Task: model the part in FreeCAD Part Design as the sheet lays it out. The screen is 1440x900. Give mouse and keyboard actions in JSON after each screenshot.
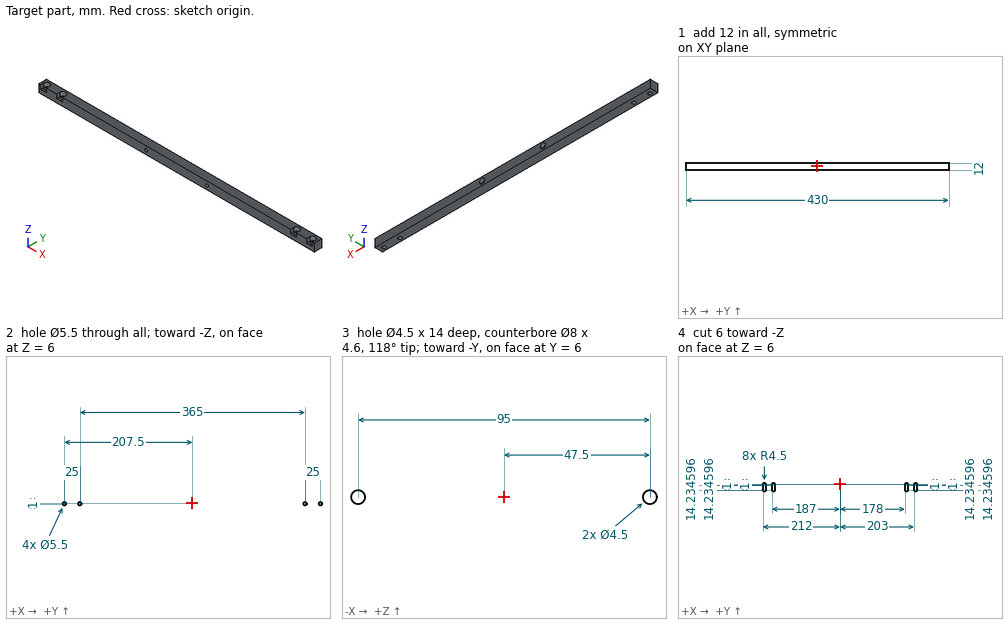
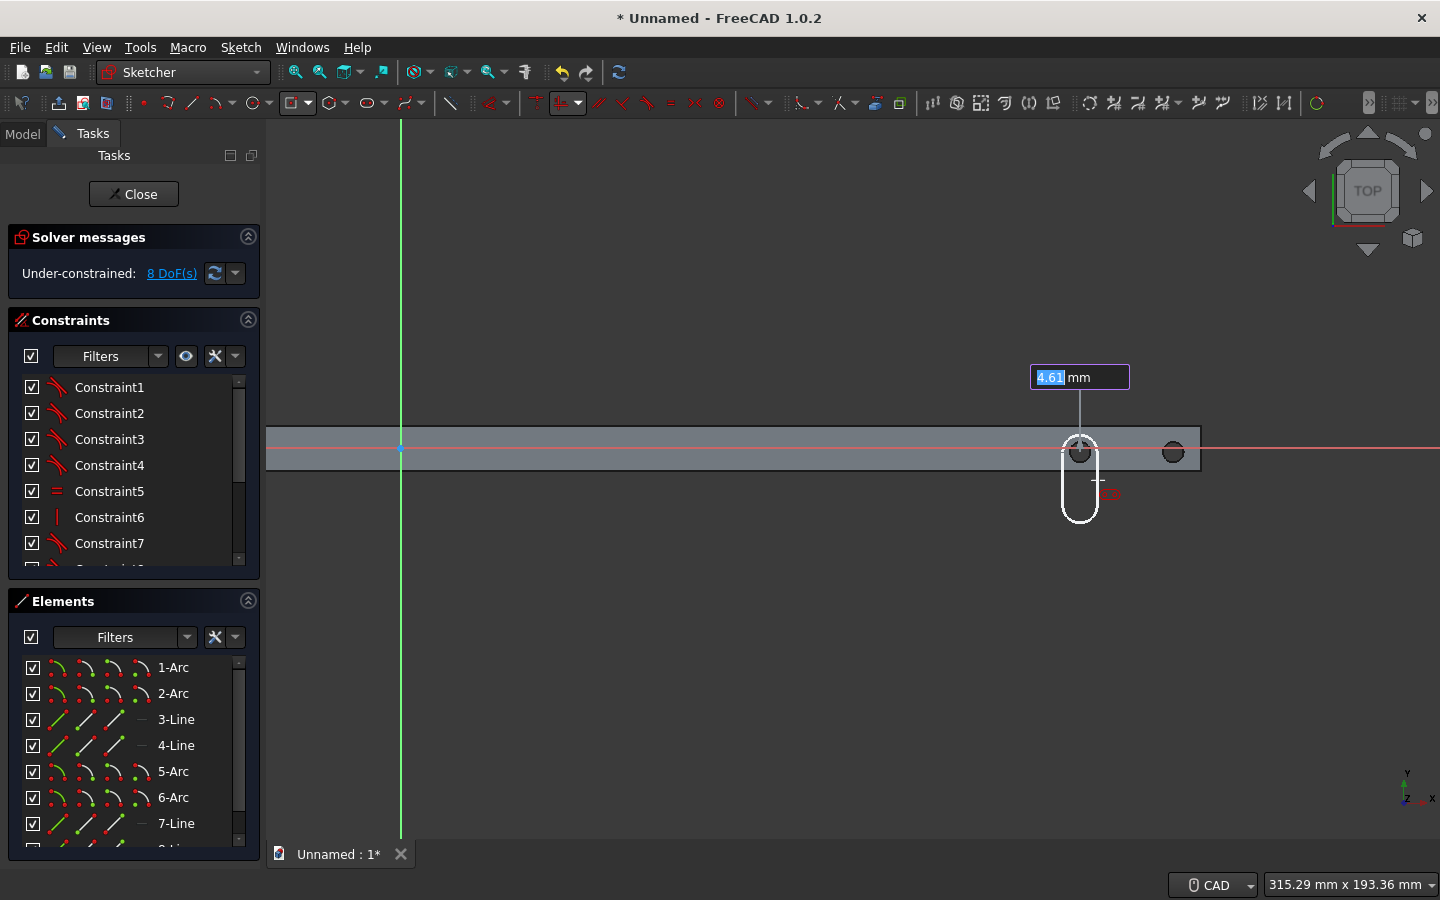
{"action": "left_click", "coordinate": [1097, 479]}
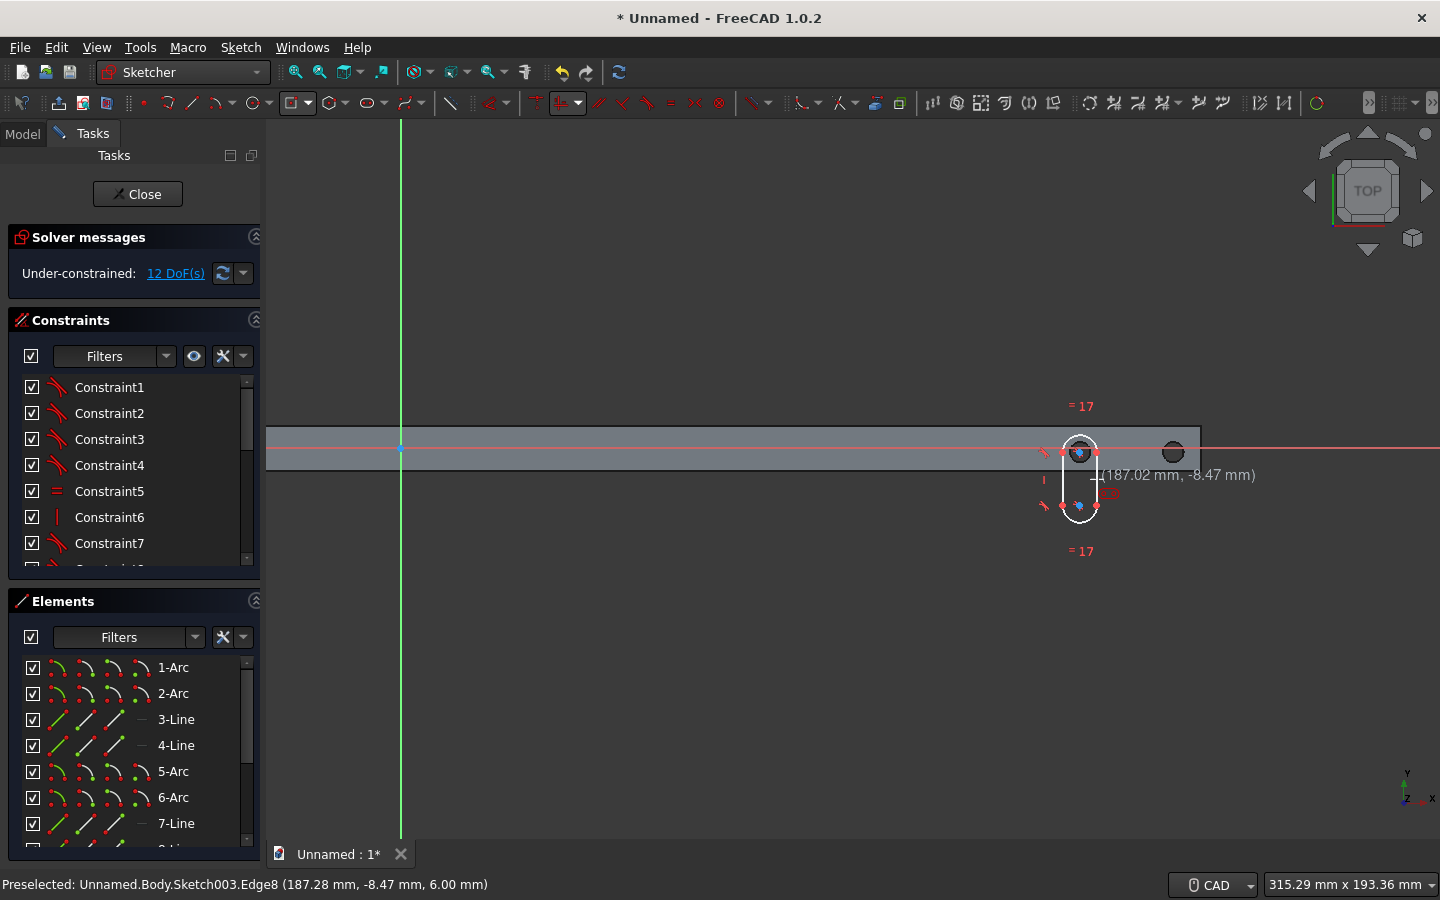
{"action": "scroll", "coordinate": [1173, 505], "scroll_direction": "up", "scroll_amount": 2}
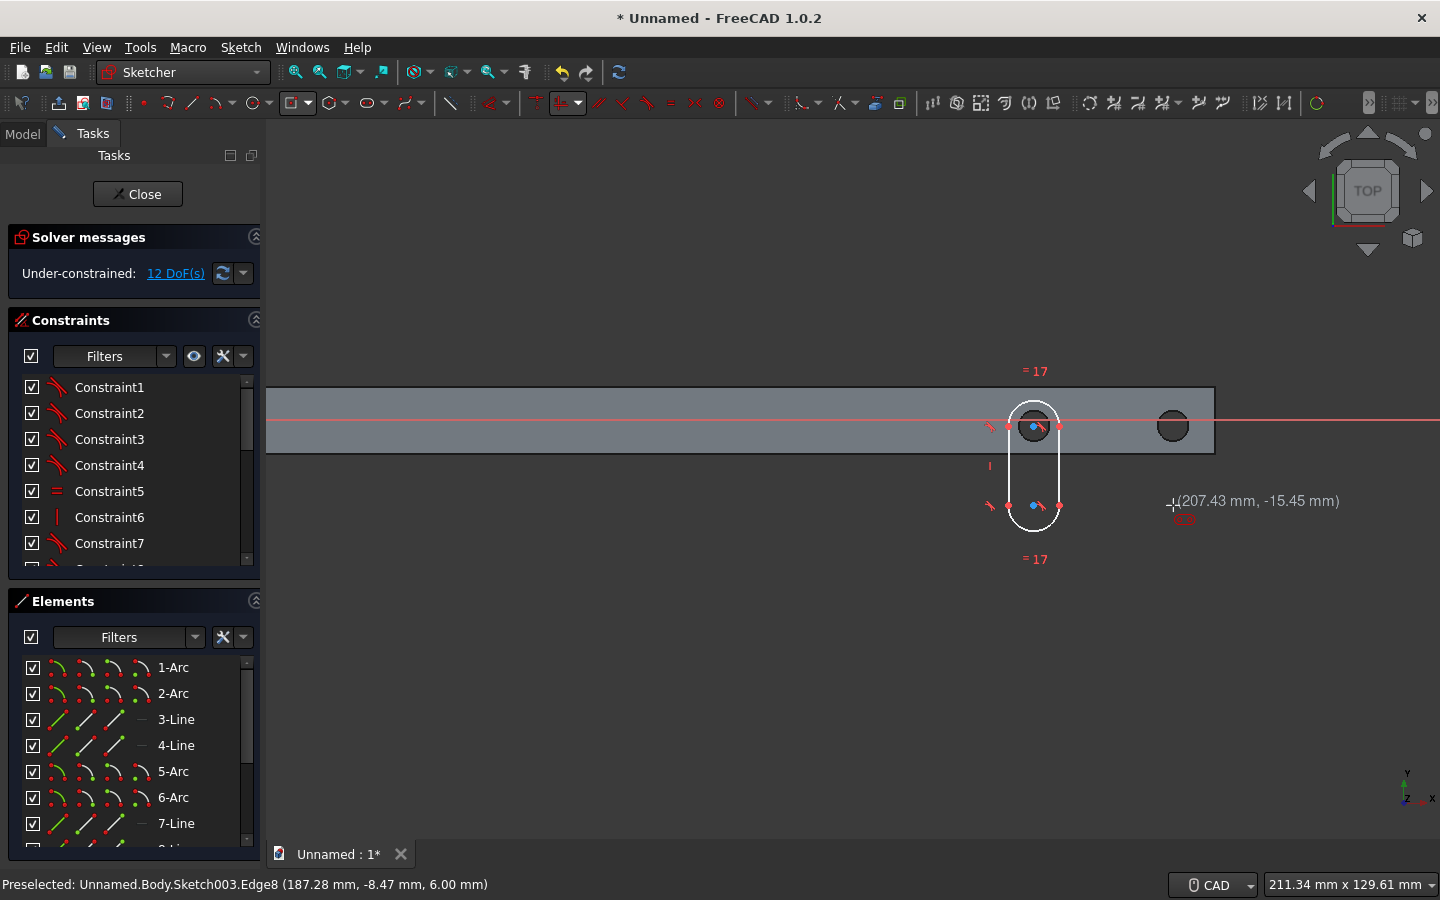
{"action": "left_click", "coordinate": [1173, 505]}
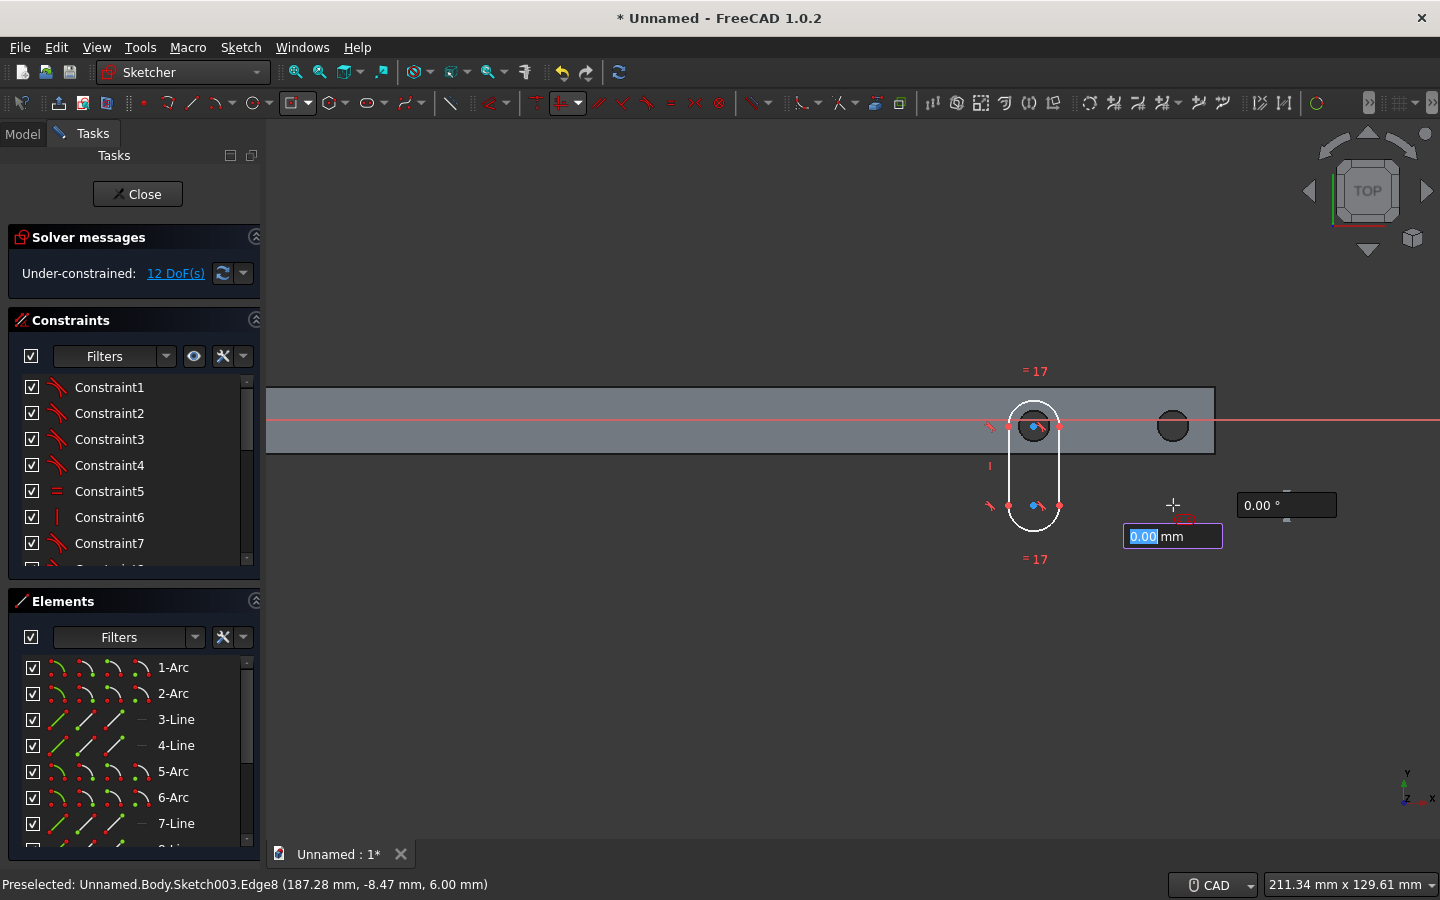
{"action": "scroll", "coordinate": [1173, 426], "scroll_direction": "up", "scroll_amount": 6}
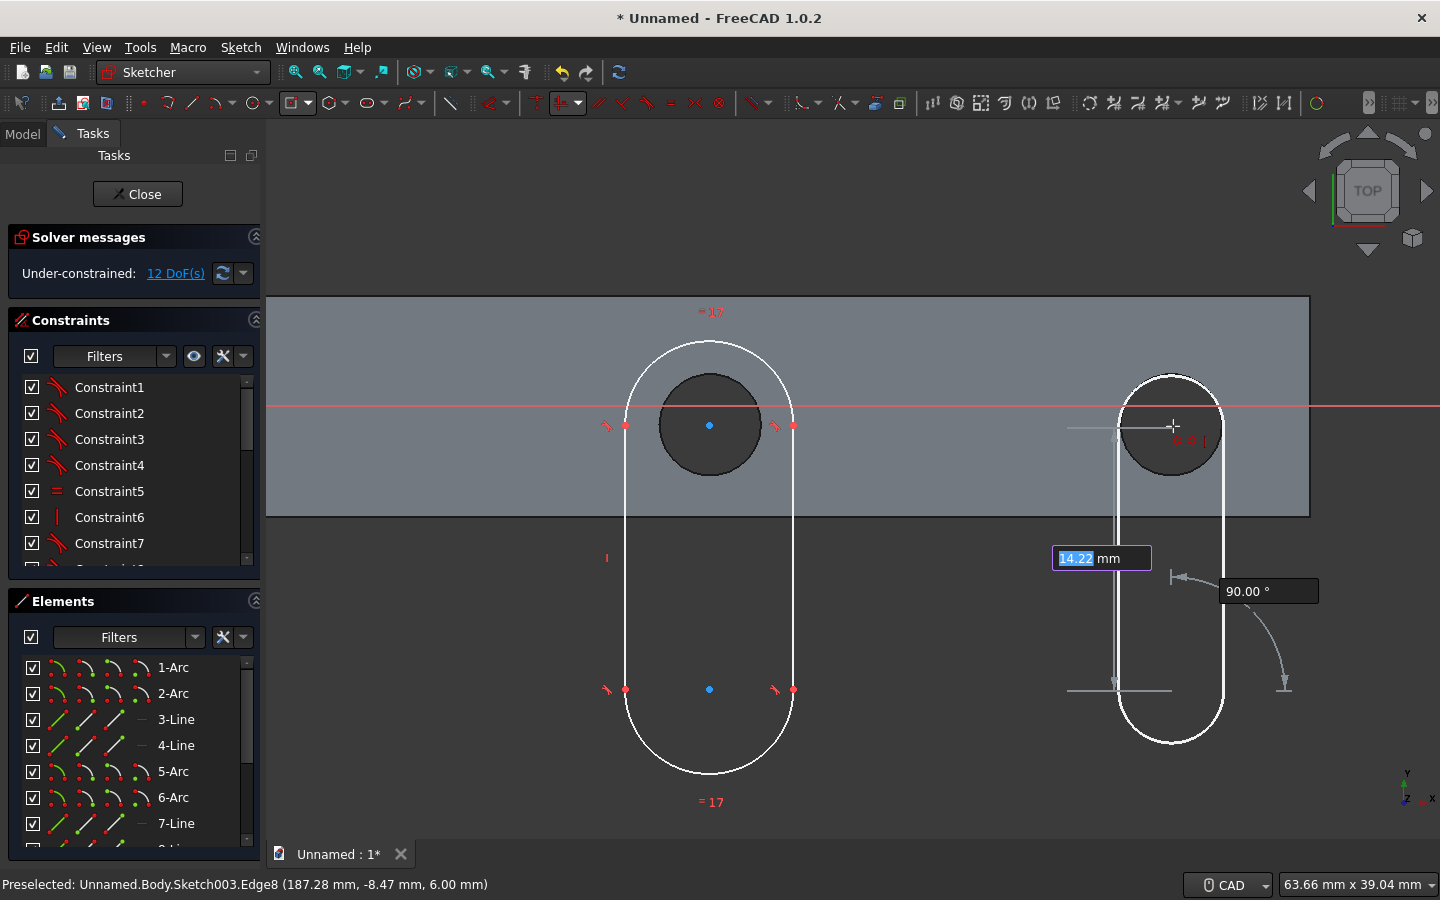
{"action": "left_click", "coordinate": [1171, 425]}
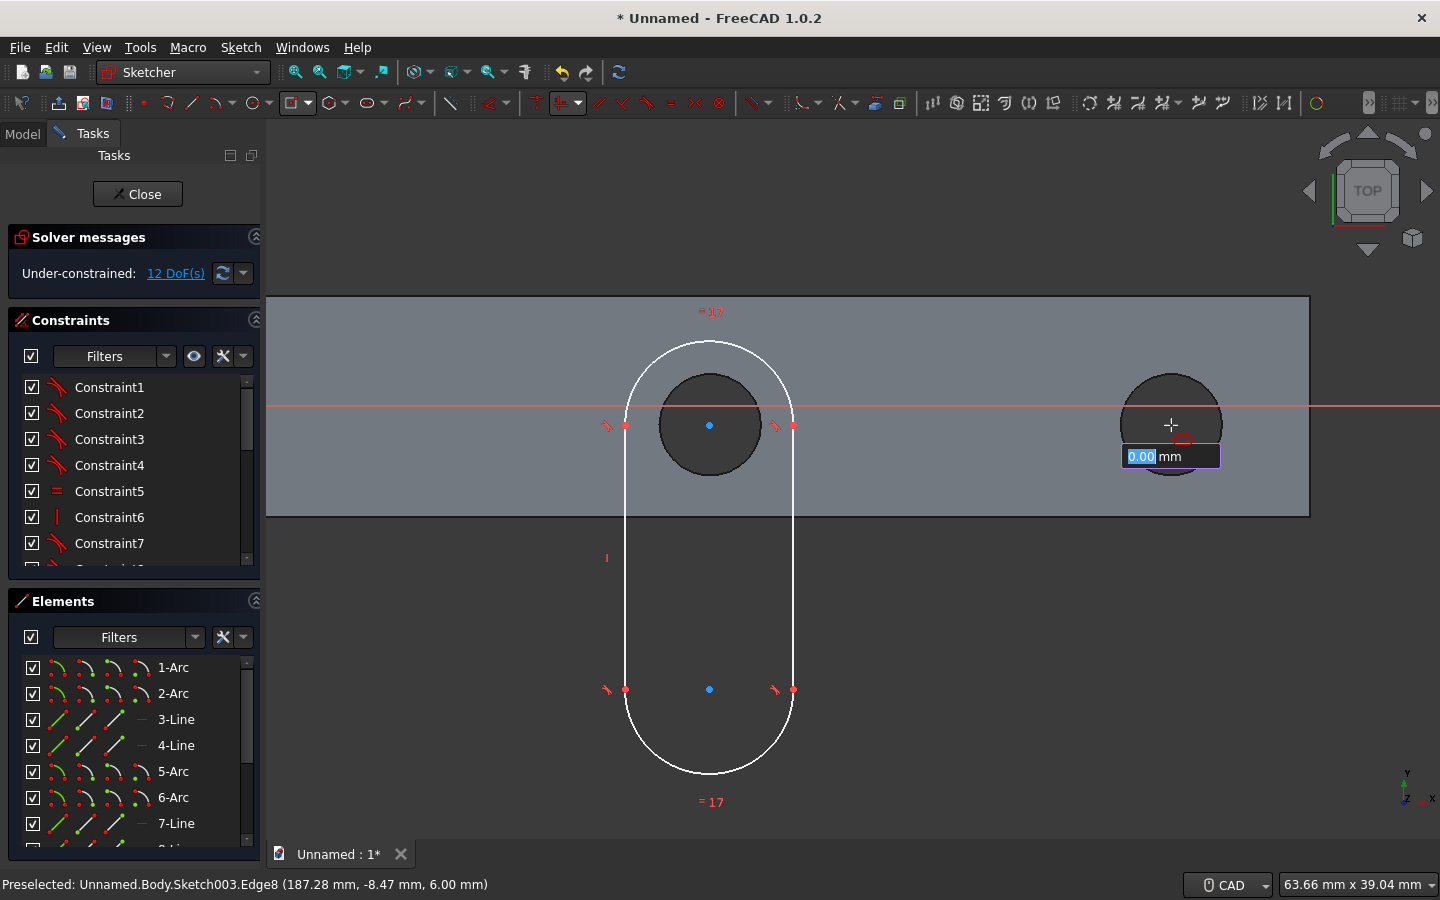
{"action": "scroll", "coordinate": [1128, 471], "scroll_direction": "down", "scroll_amount": 12}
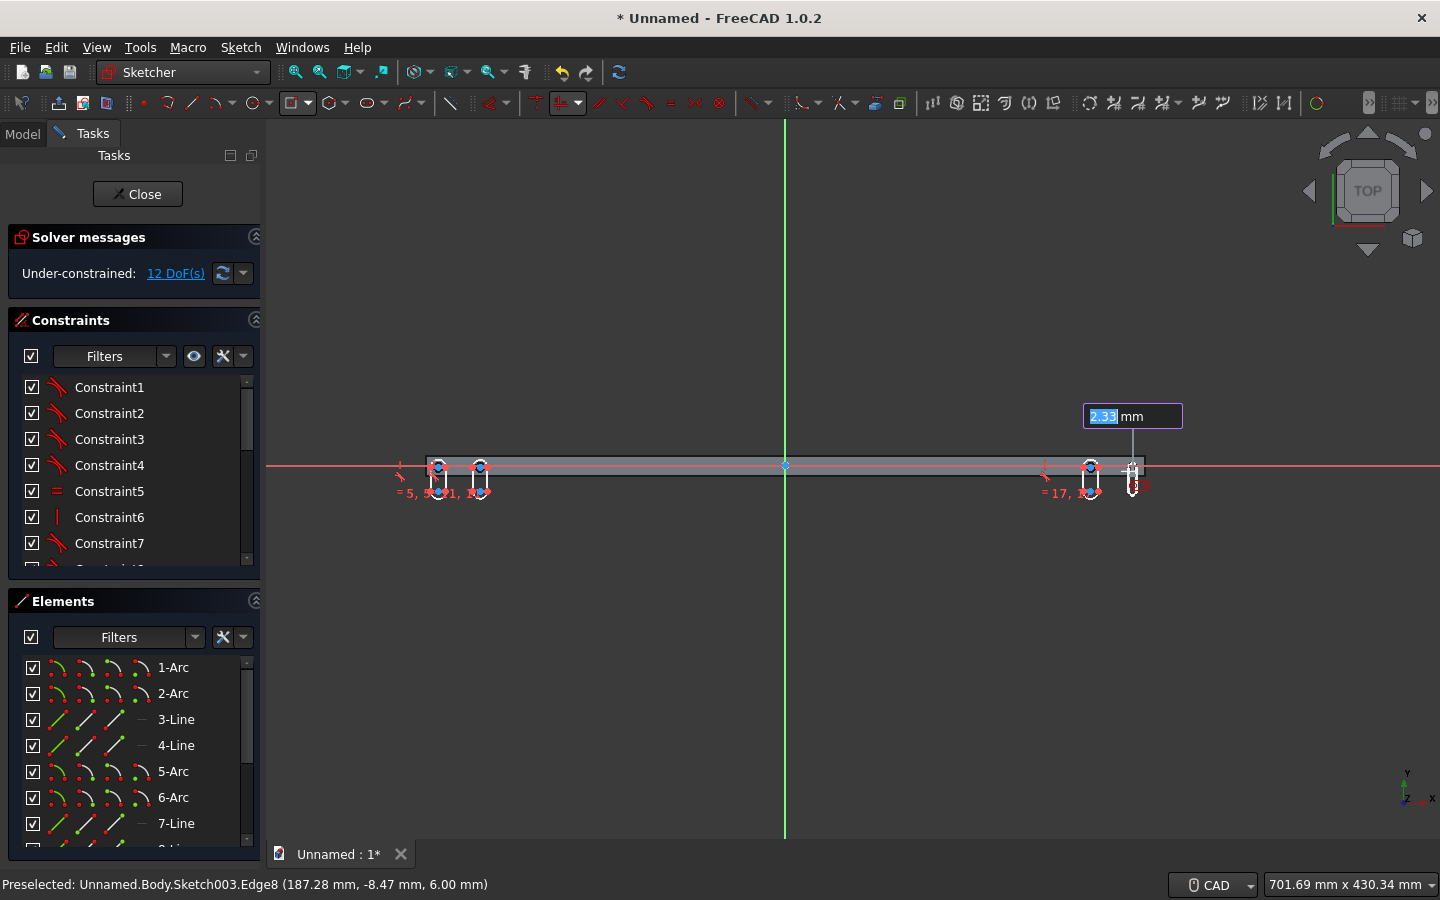
{"action": "scroll", "coordinate": [1140, 479], "scroll_direction": "up", "scroll_amount": 4}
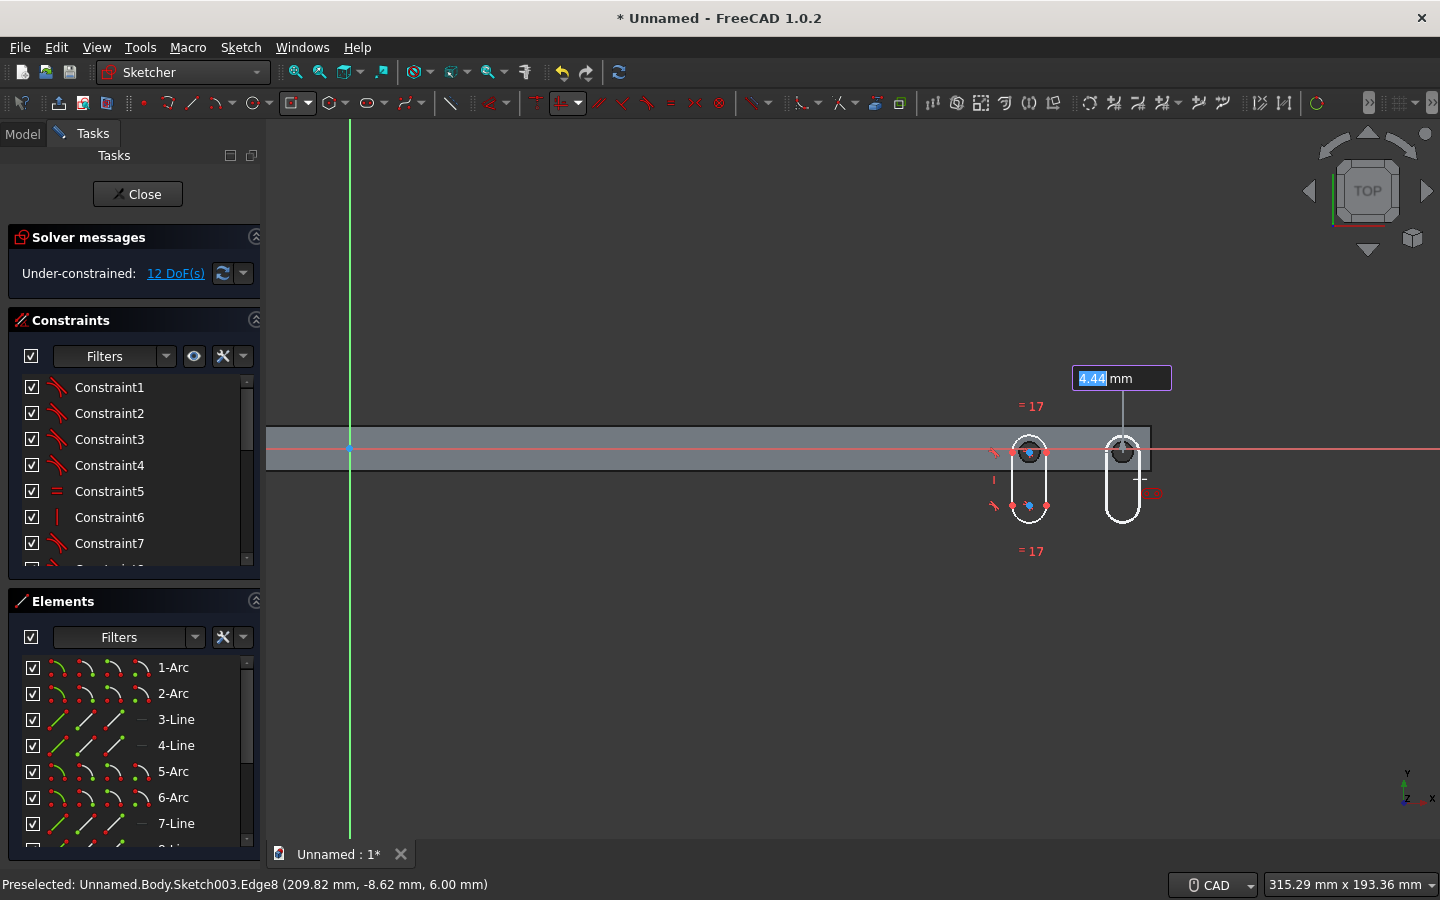
{"action": "left_click", "coordinate": [1139, 479]}
{"action": "key", "text": "Escape"}